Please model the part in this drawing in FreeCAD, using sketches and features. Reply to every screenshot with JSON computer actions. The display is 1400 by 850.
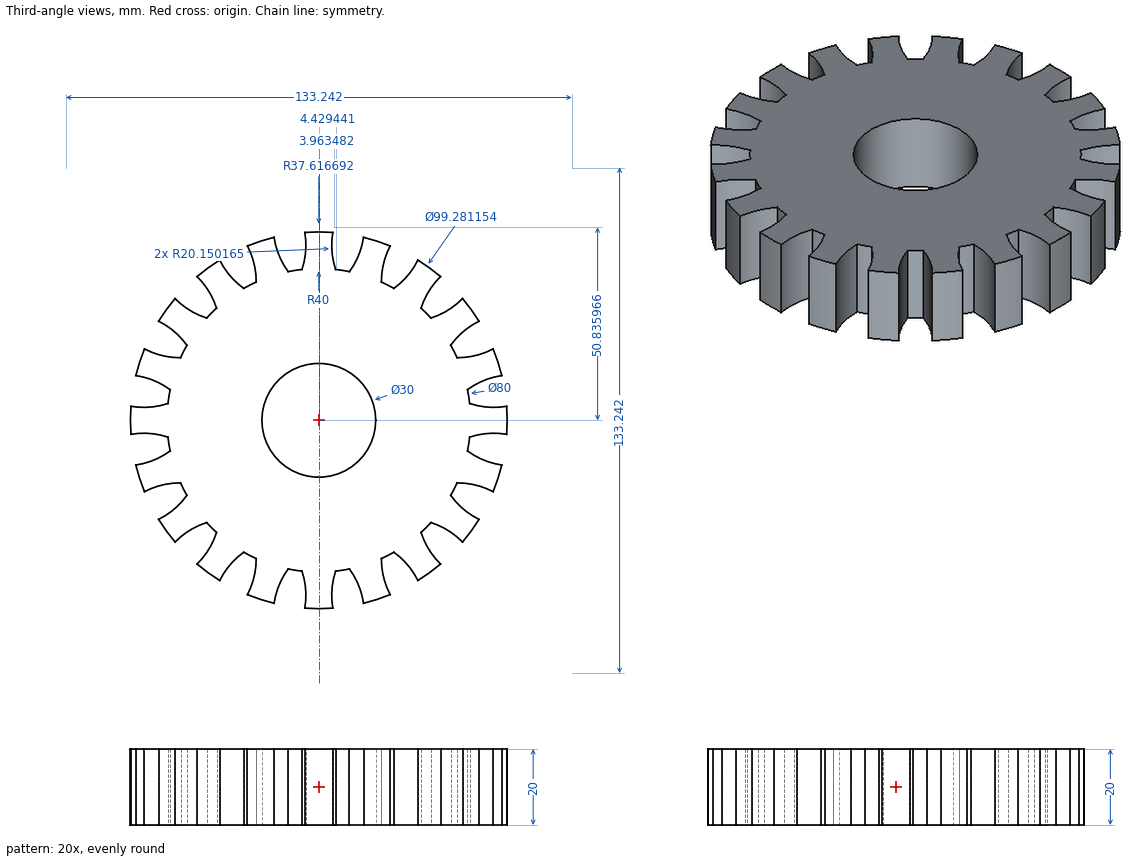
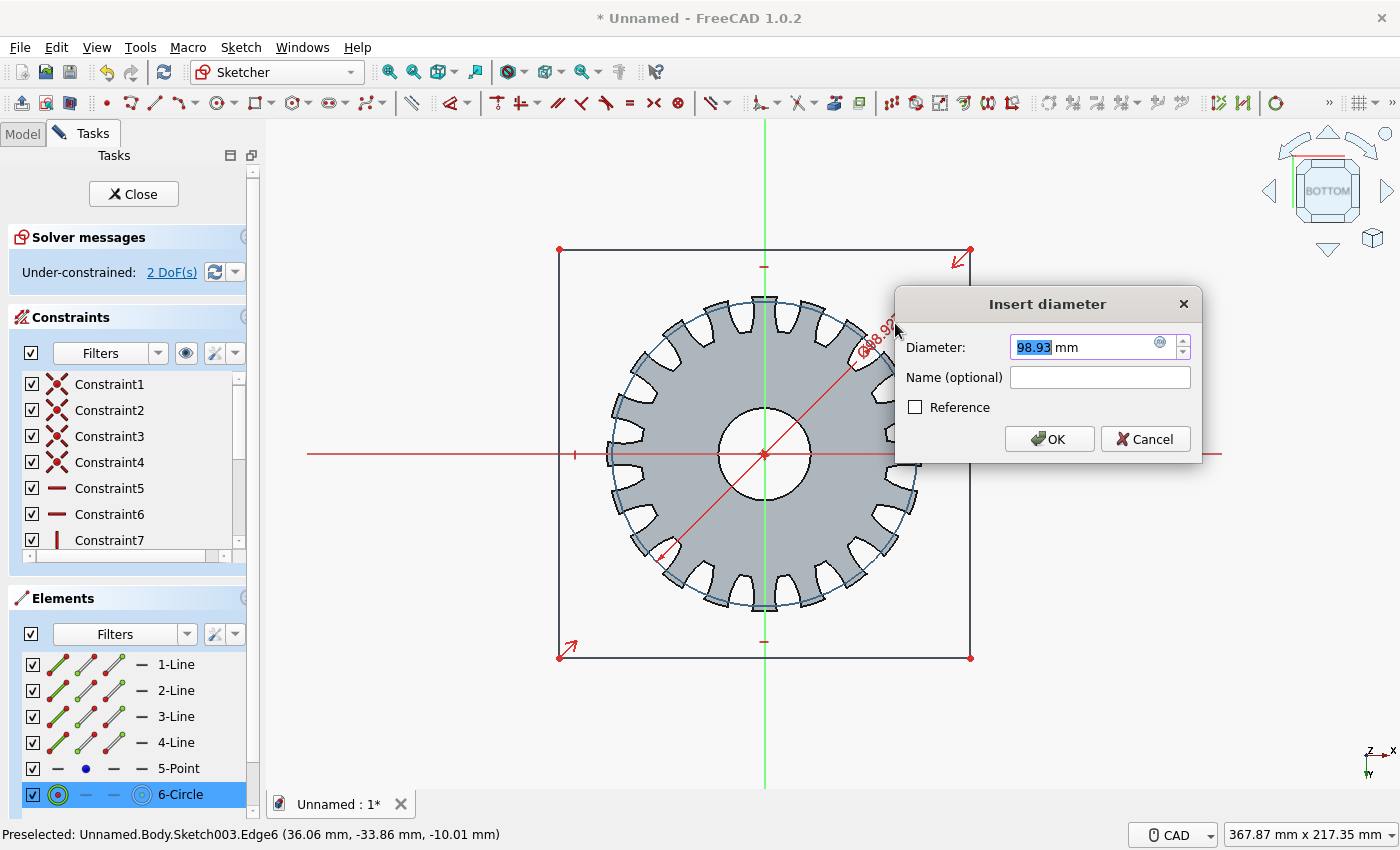
{"action": "type", "text": "99.281154"}
{"action": "key", "text": "Return"}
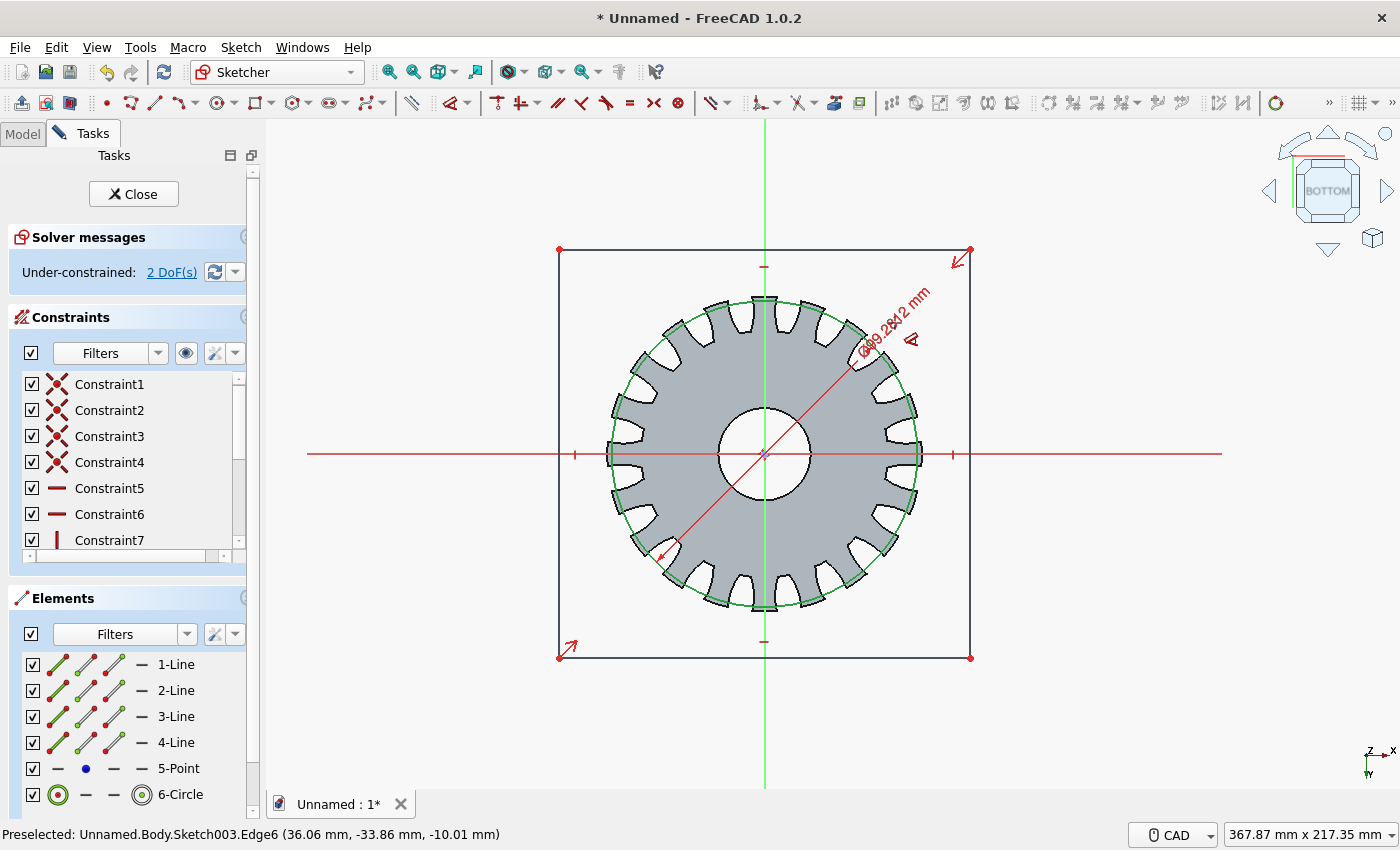
{"action": "left_click", "coordinate": [682, 658]}
{"action": "left_click", "coordinate": [670, 692]}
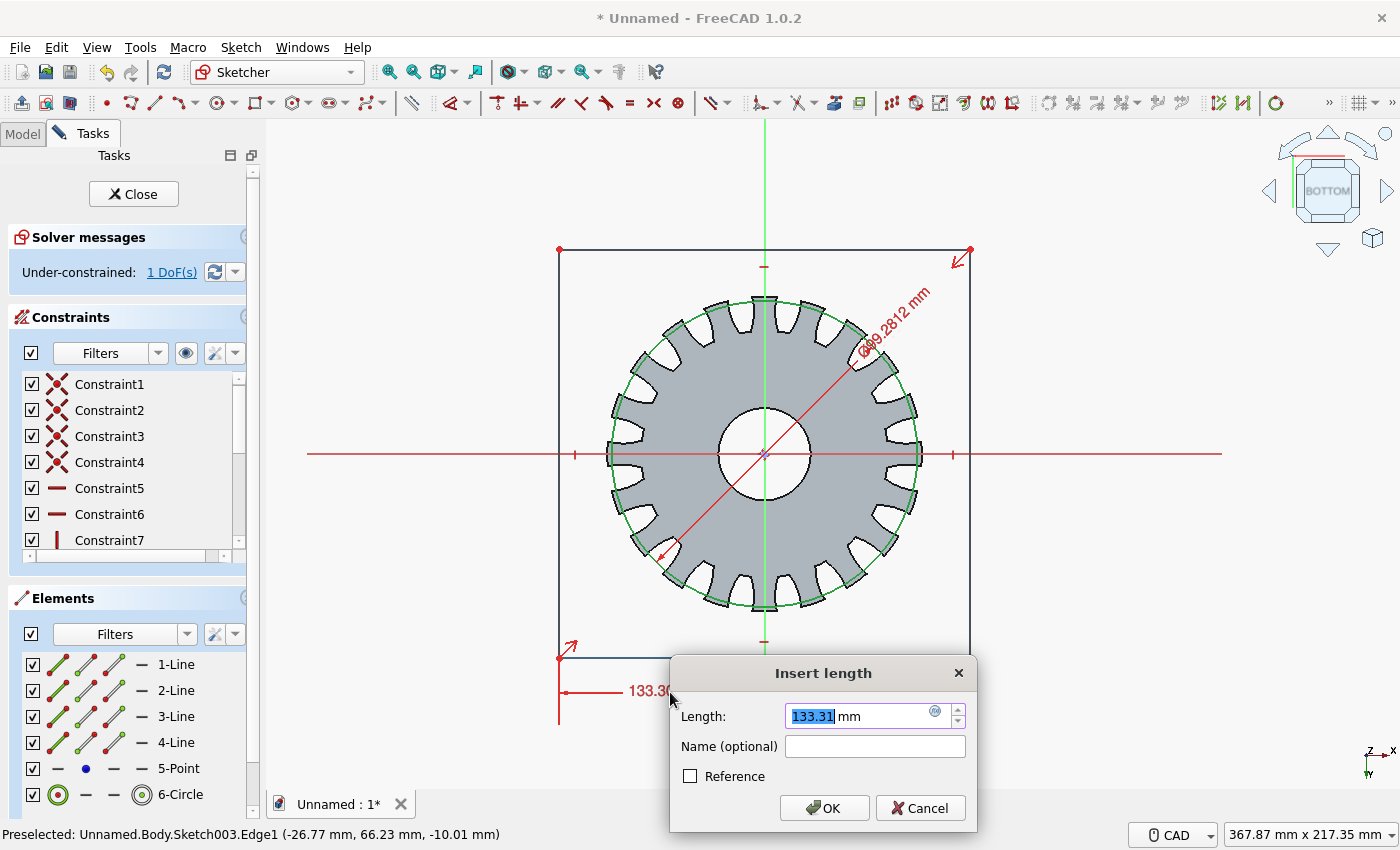
{"action": "type", "text": "133.242"}
{"action": "key", "text": "Return"}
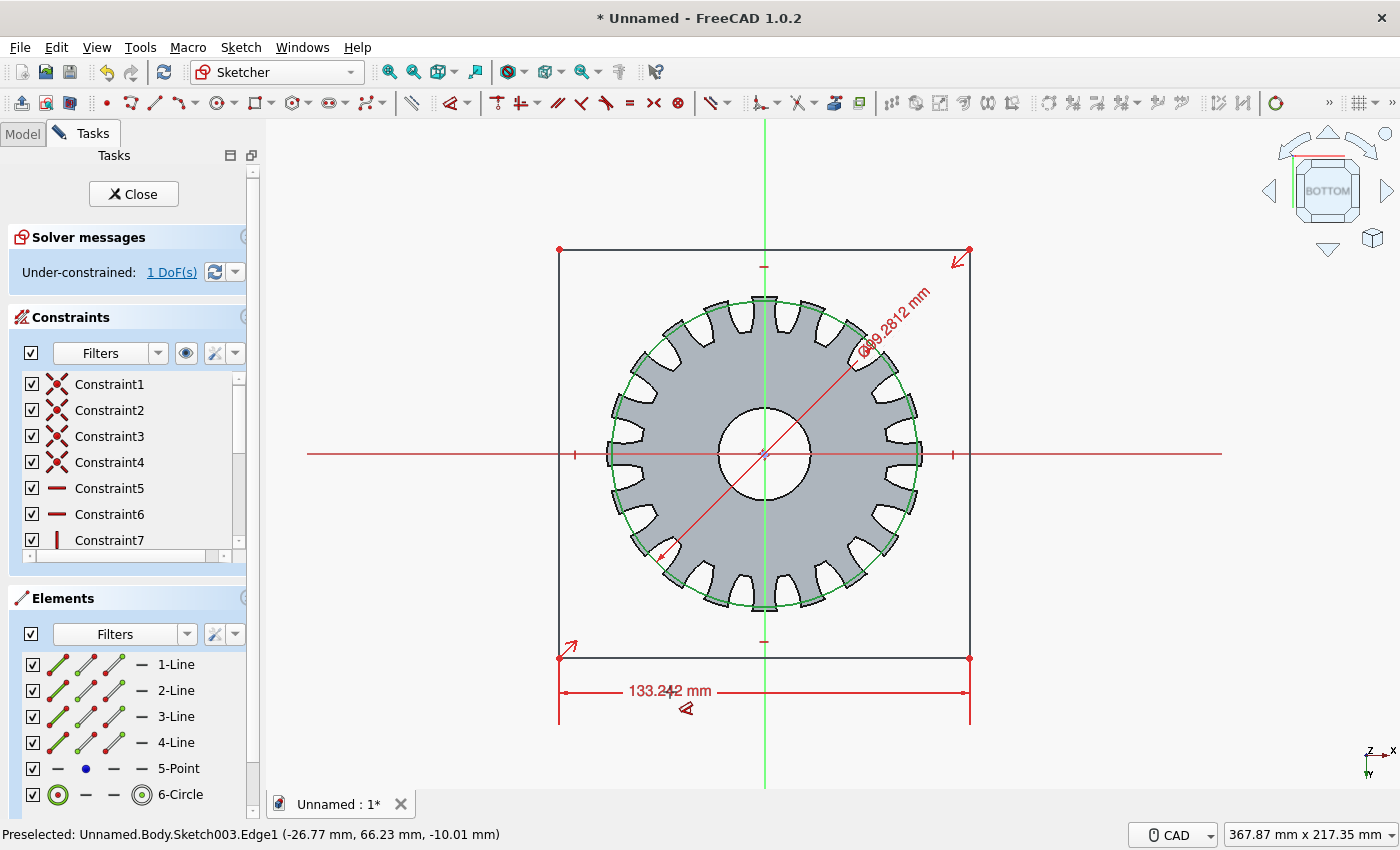
{"action": "left_click", "coordinate": [970, 536]}
{"action": "left_click", "coordinate": [1004, 360]}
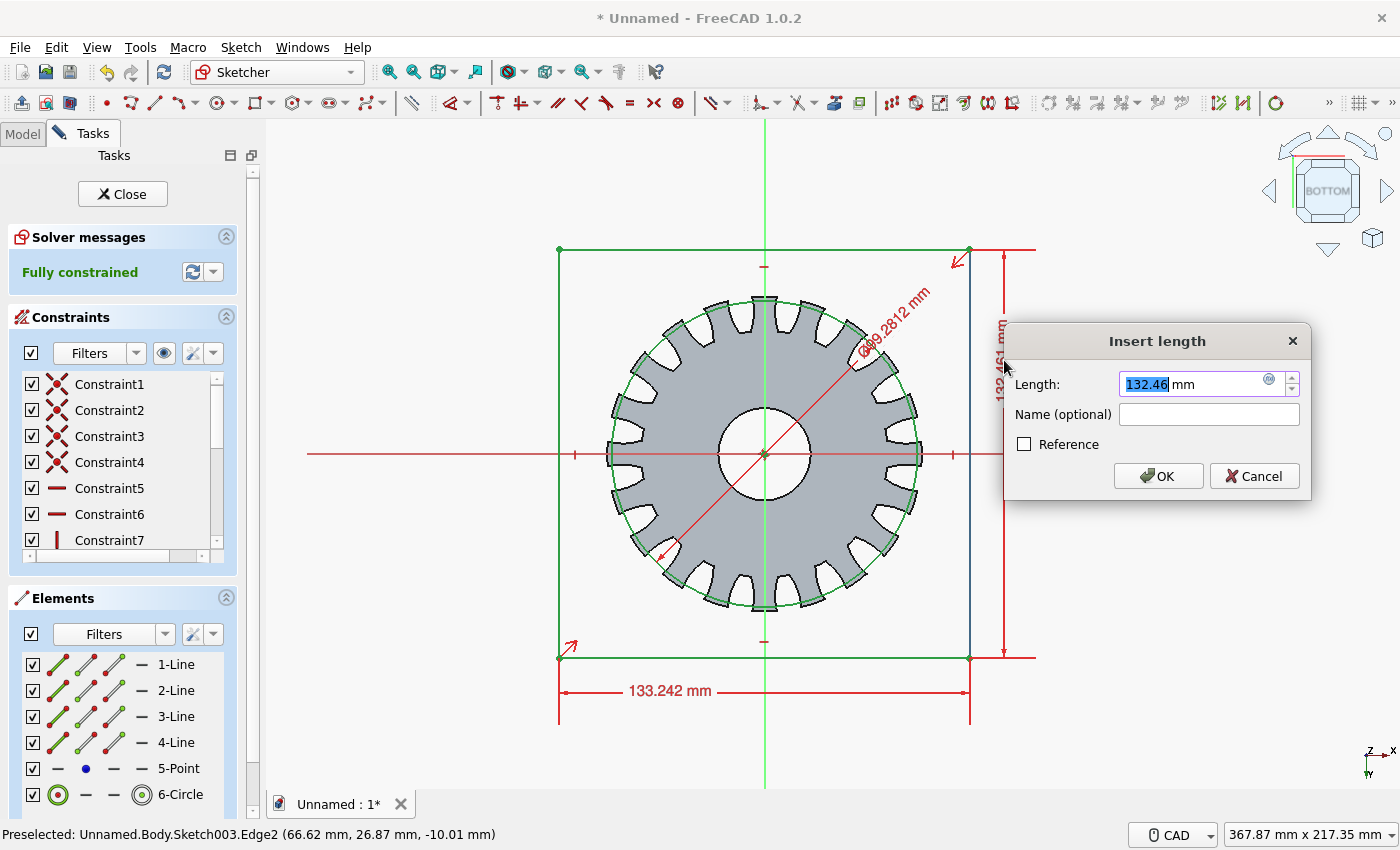
{"action": "type", "text": "133.242"}
{"action": "key", "text": "Return"}
{"action": "key", "text": "Escape"}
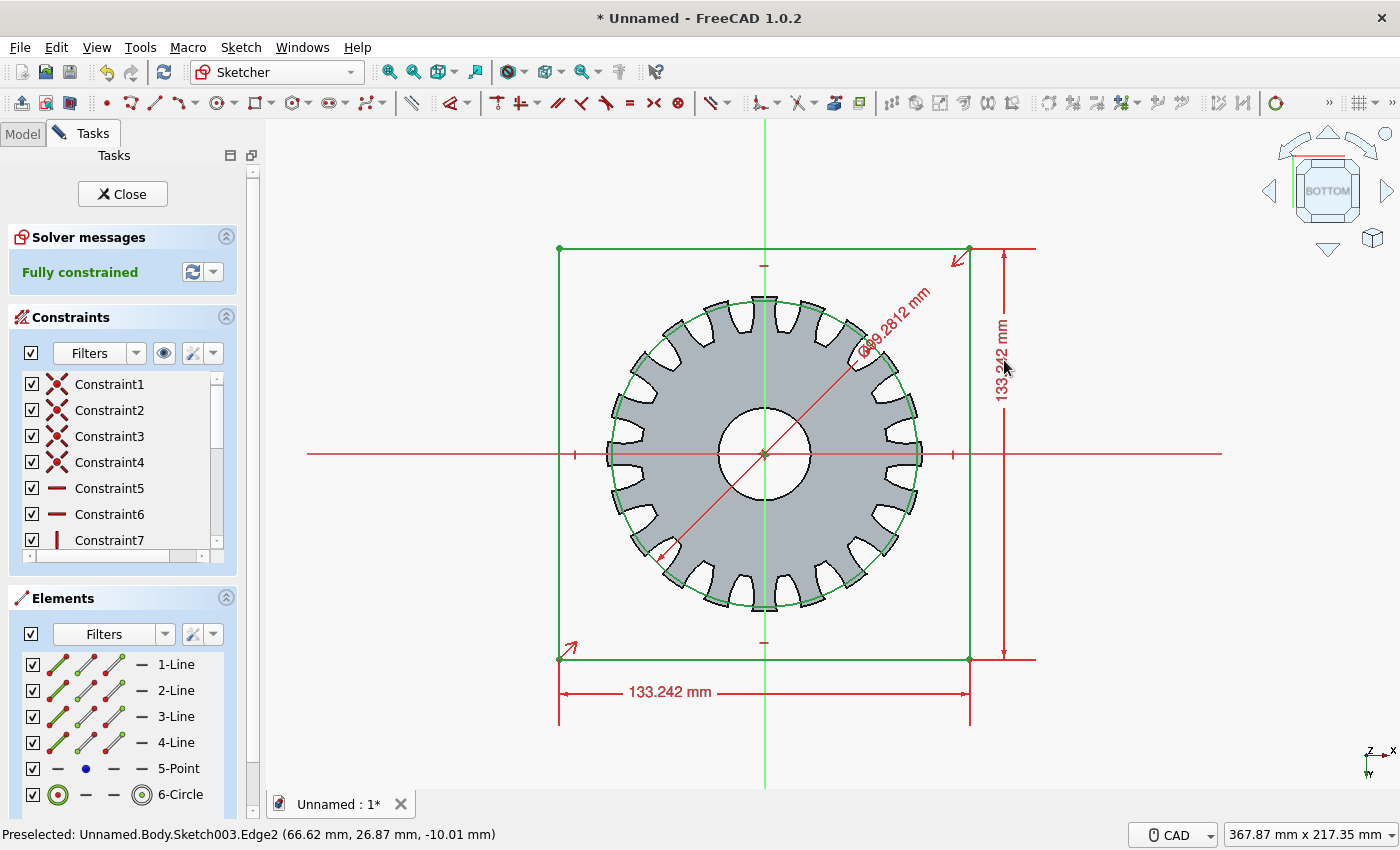
{"action": "left_click", "coordinate": [123, 194]}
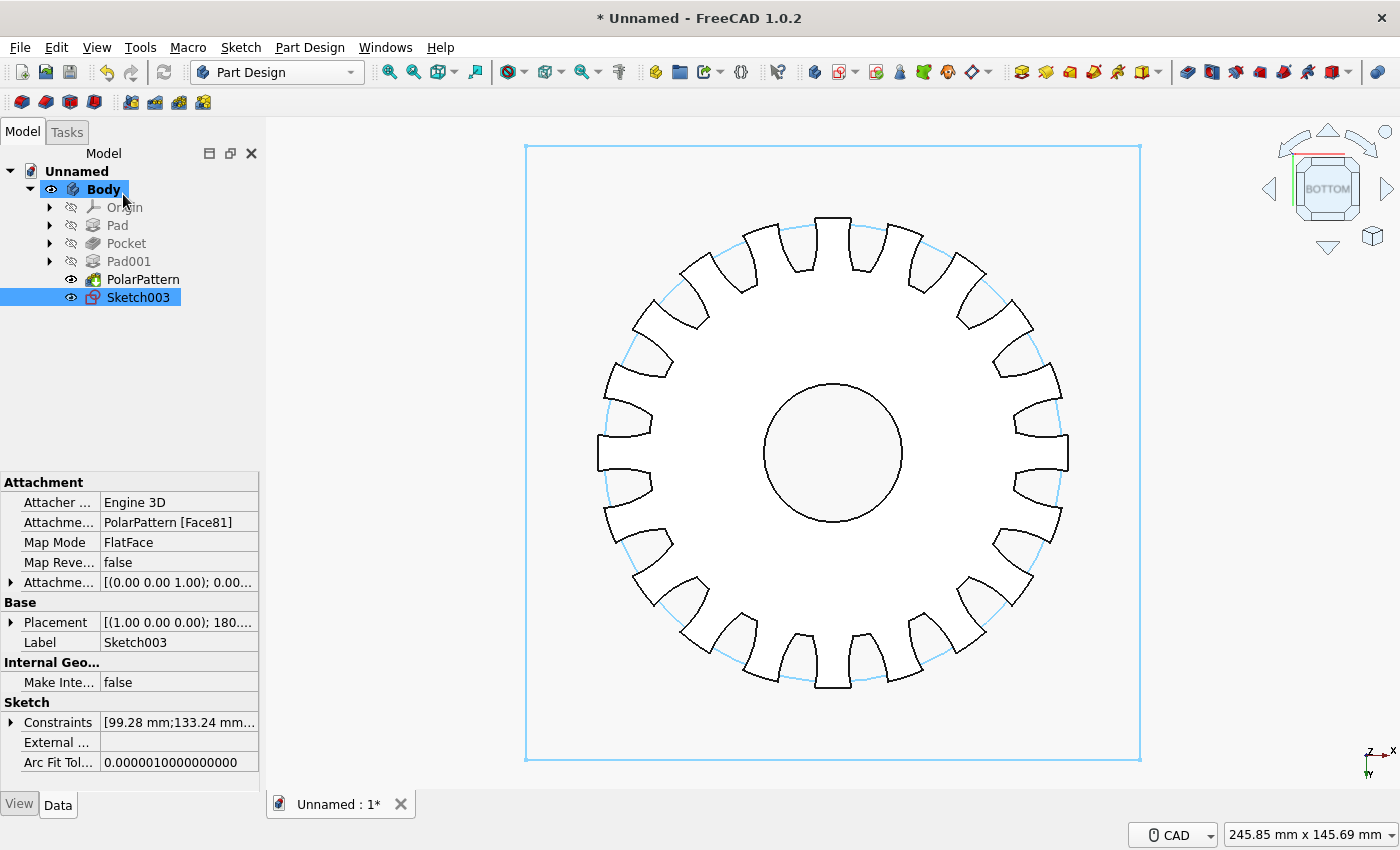
{"action": "left_click", "coordinate": [1188, 72]}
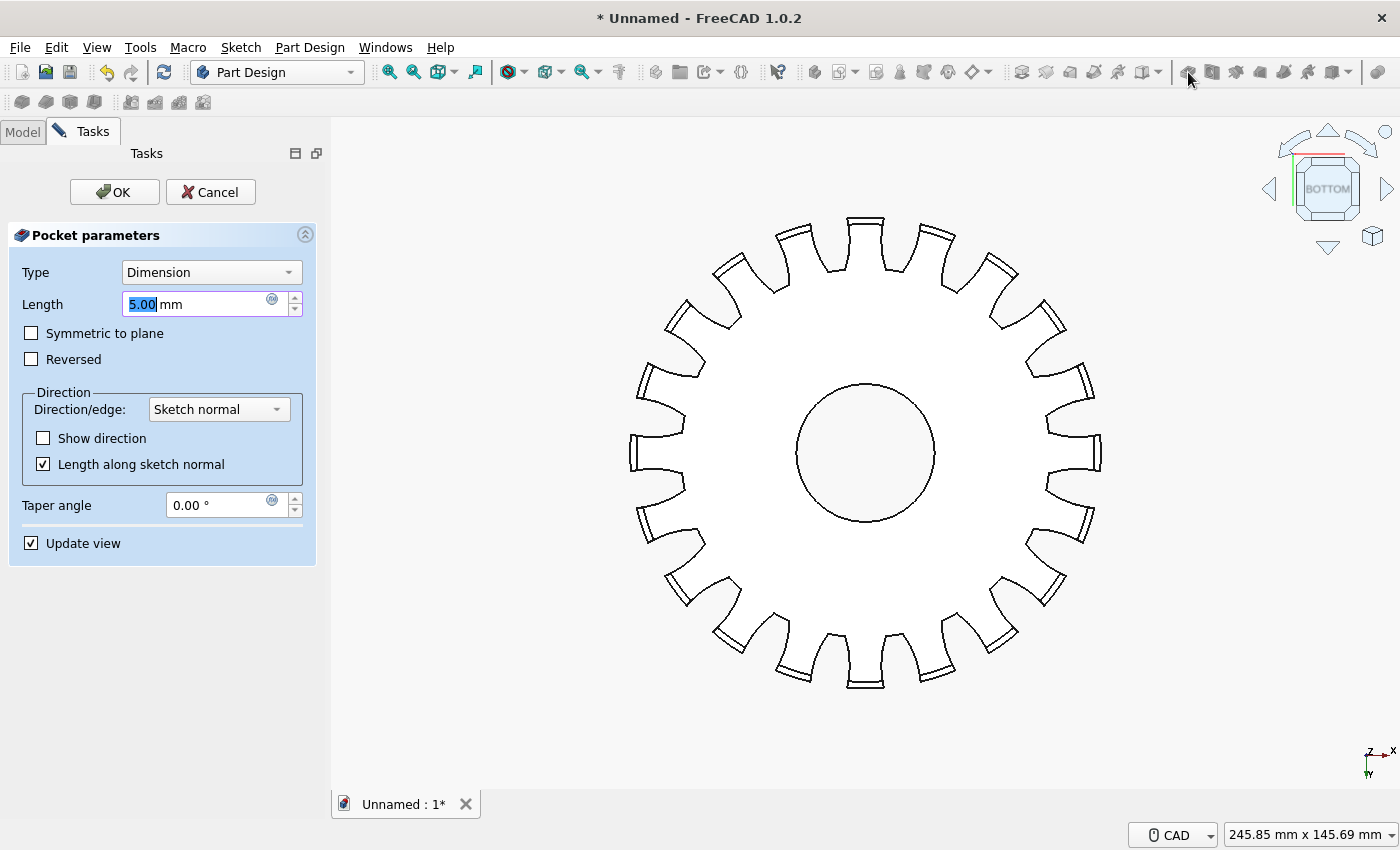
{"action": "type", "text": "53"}
{"action": "key", "text": "Tab"}